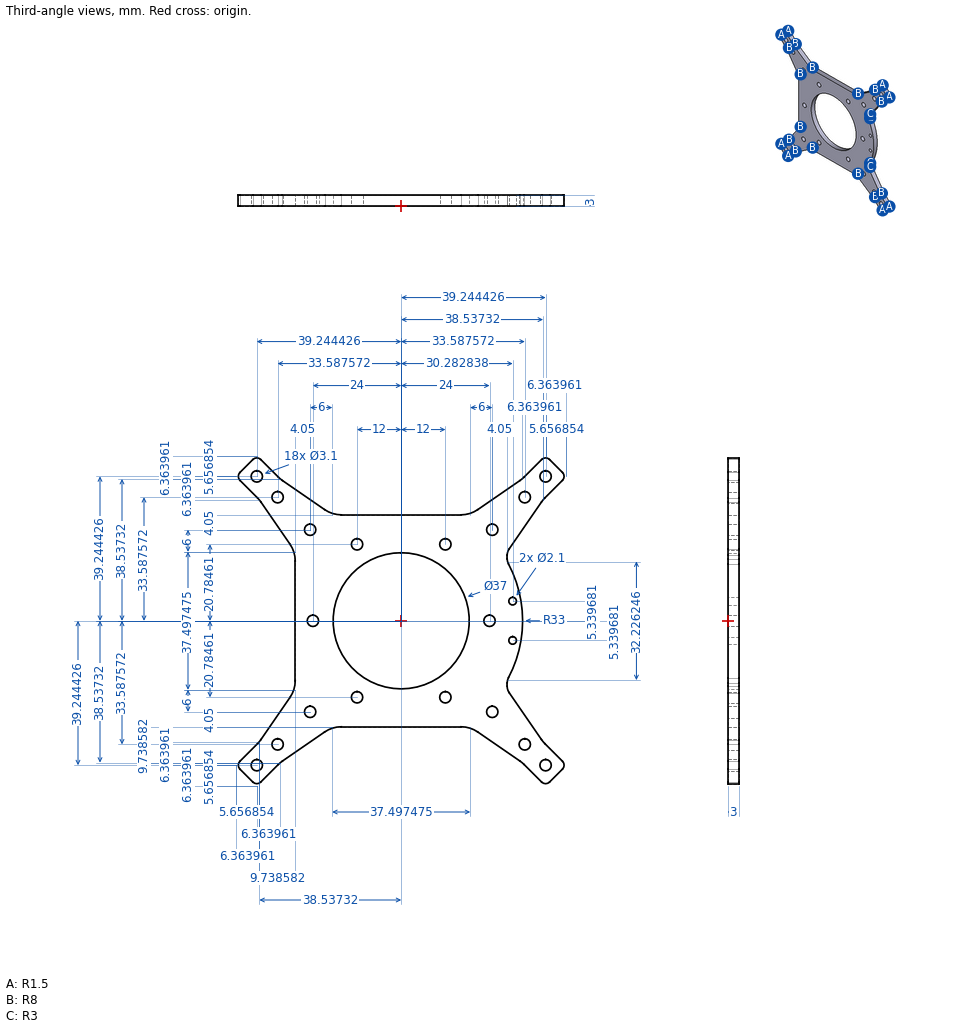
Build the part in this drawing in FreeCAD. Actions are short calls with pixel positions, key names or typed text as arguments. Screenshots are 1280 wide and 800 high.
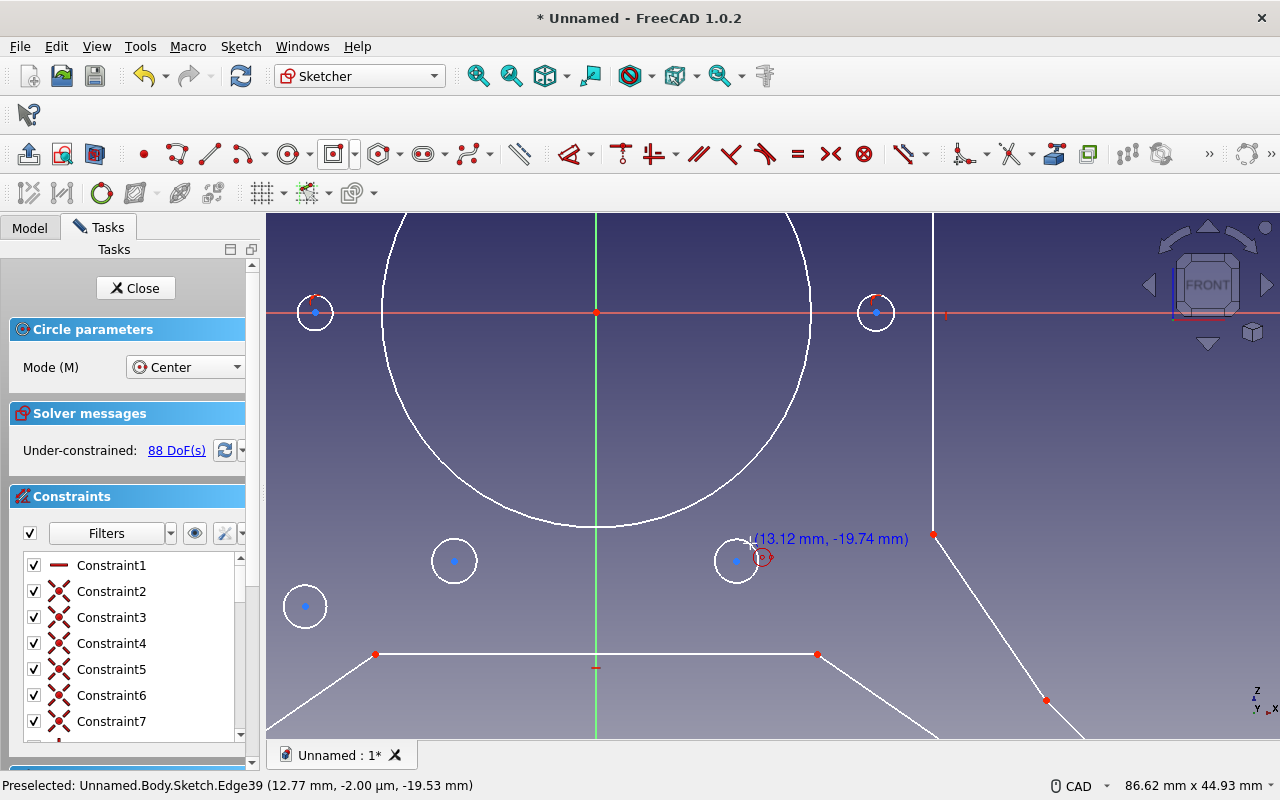
scroll(886, 603, up, 2)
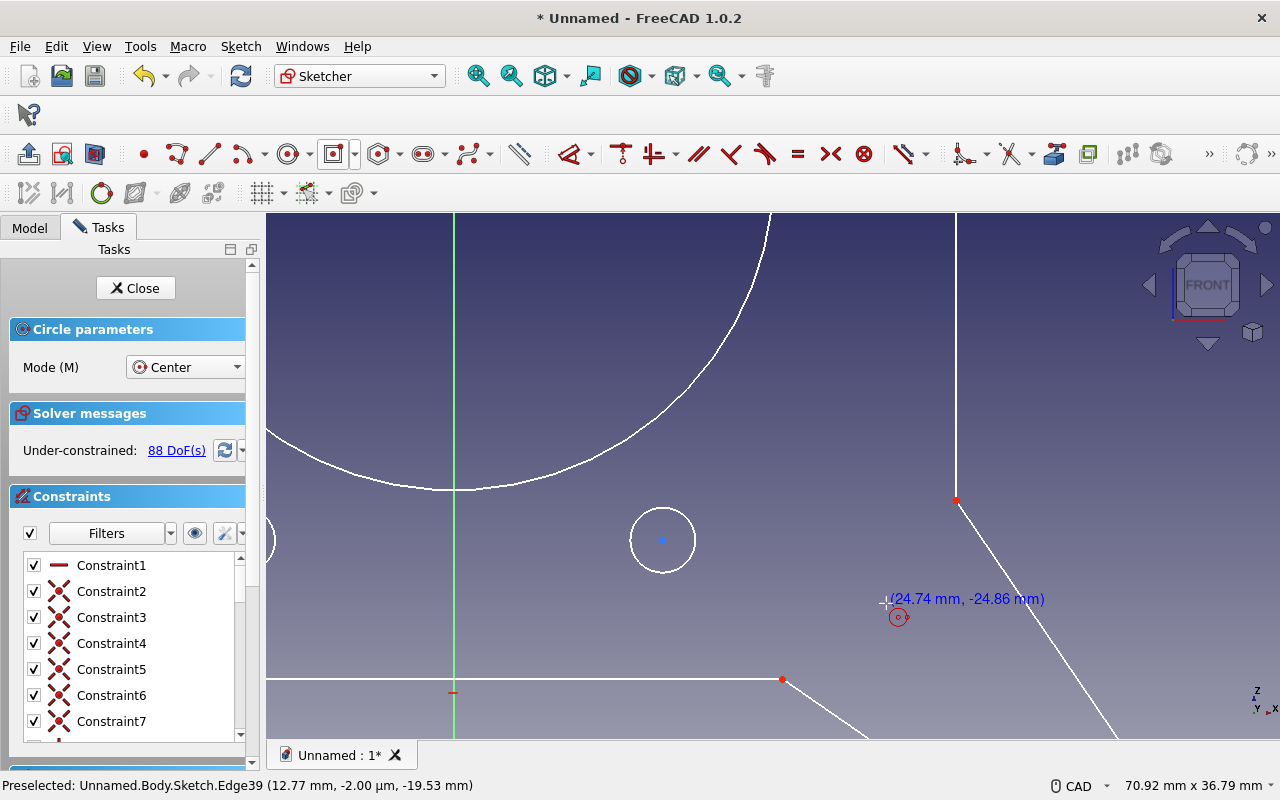
scroll(768, 553, down, 8)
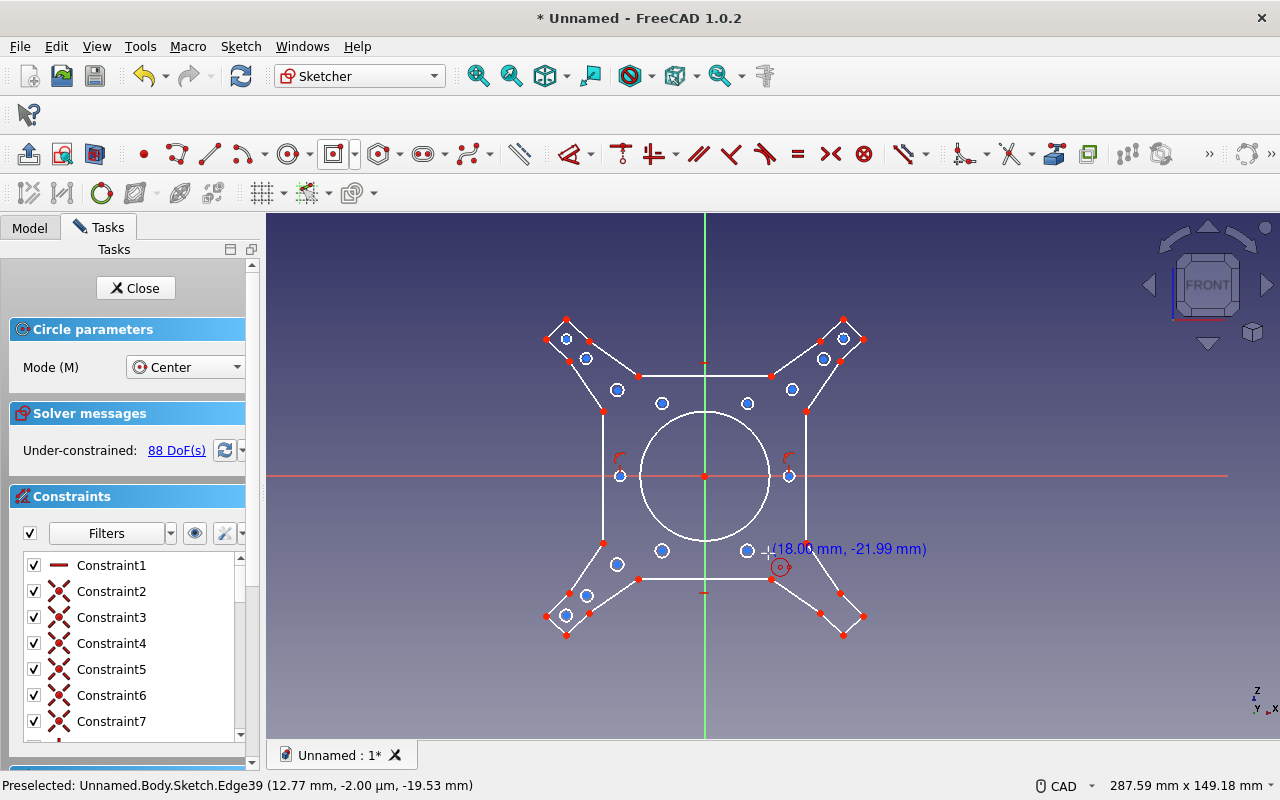
click(792, 563)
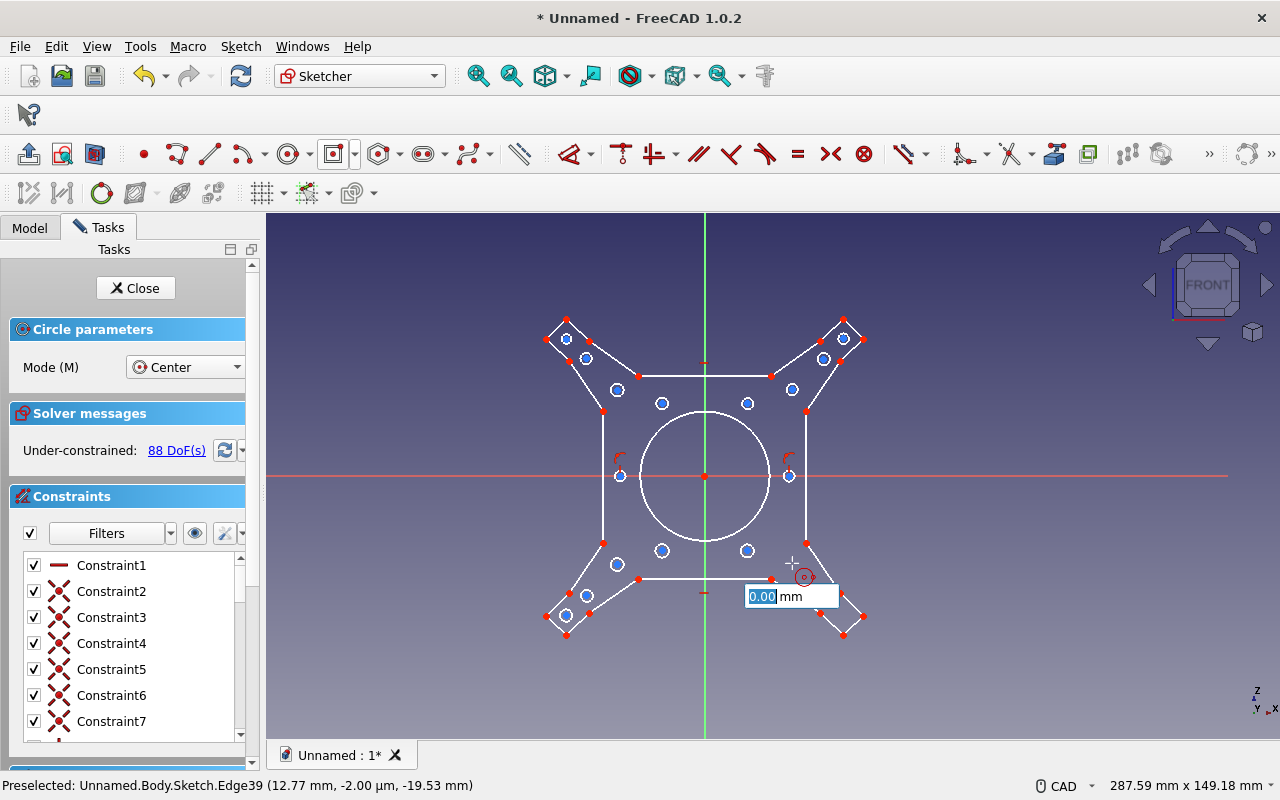
scroll(796, 560, up, 6)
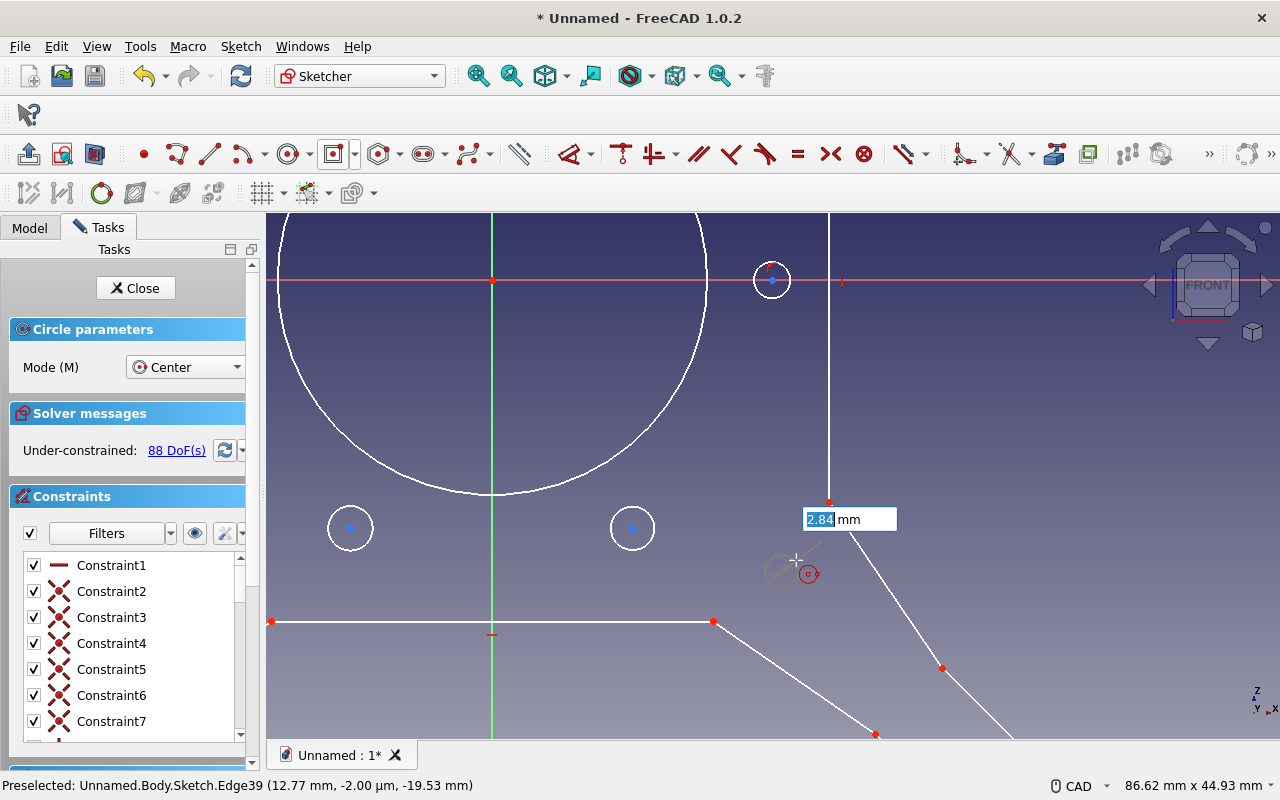
click(795, 557)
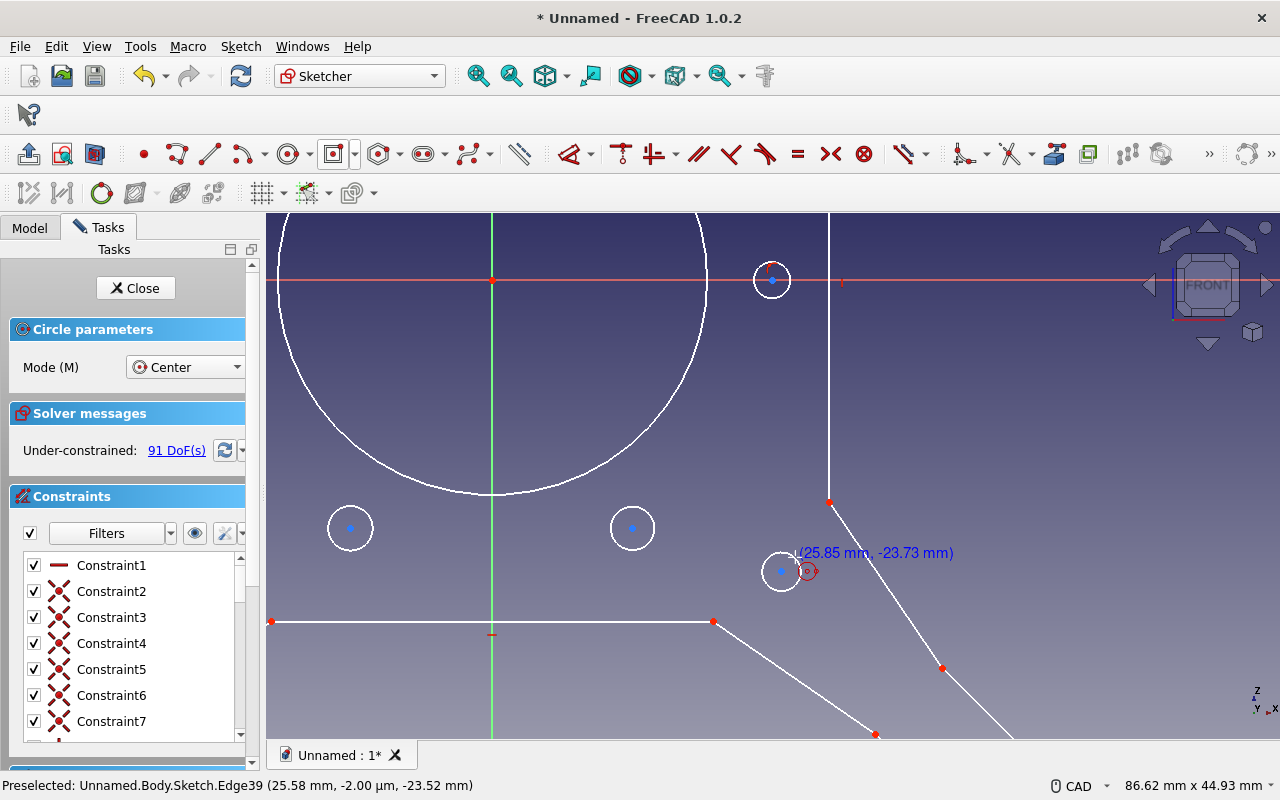
scroll(886, 673, up, 2)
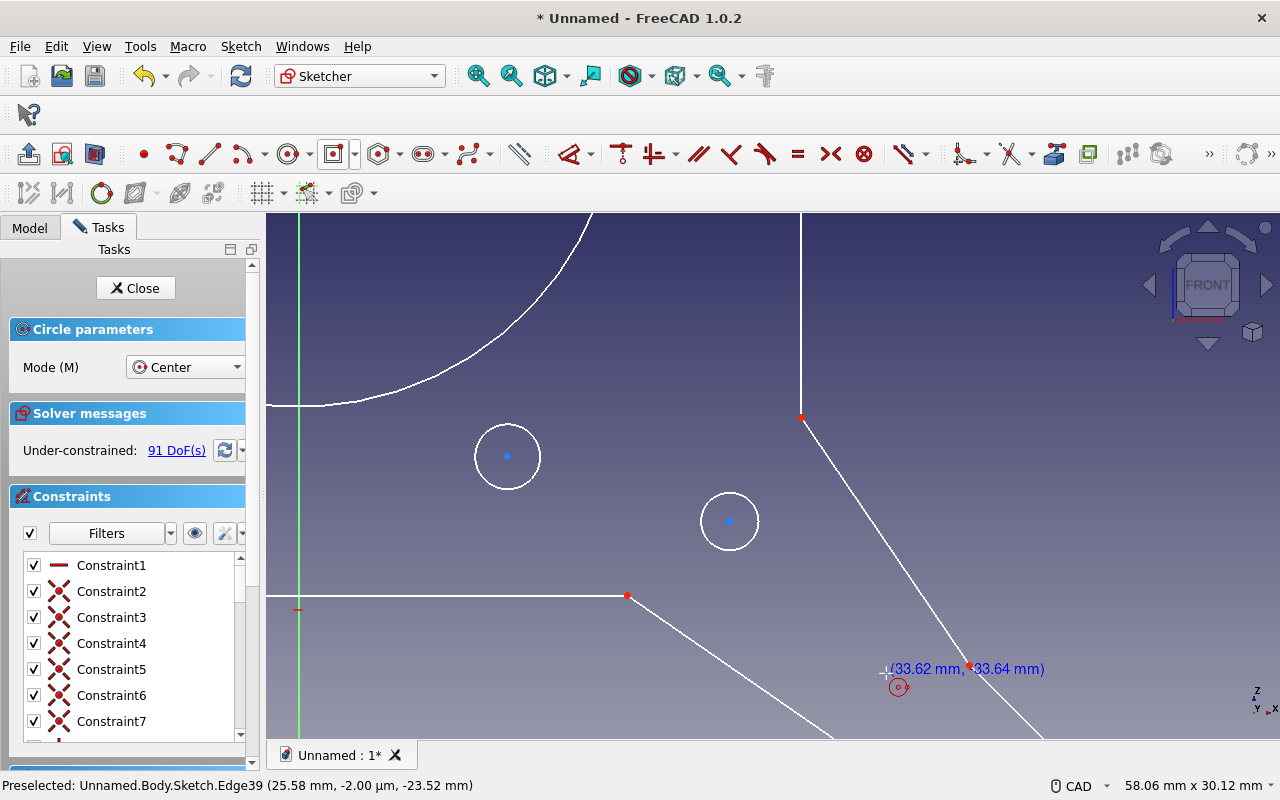
scroll(807, 575, down, 8)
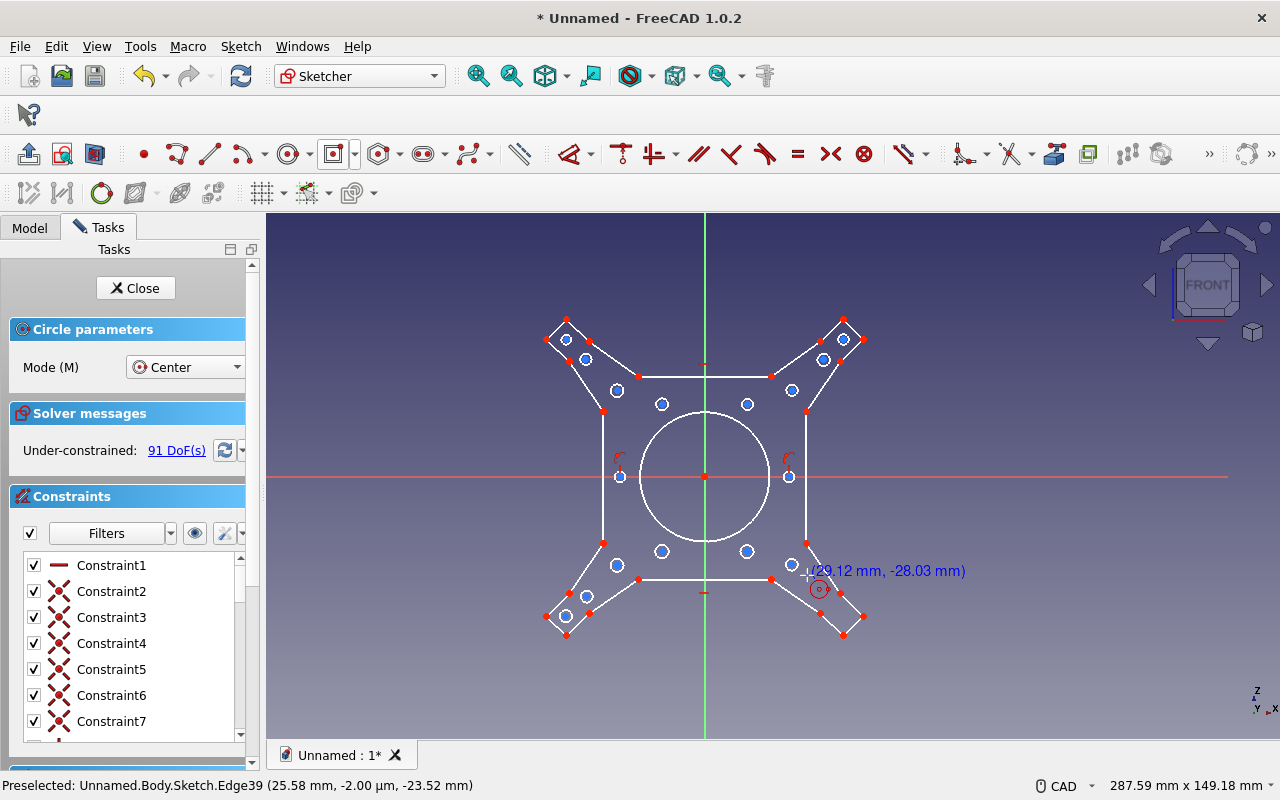
click(823, 595)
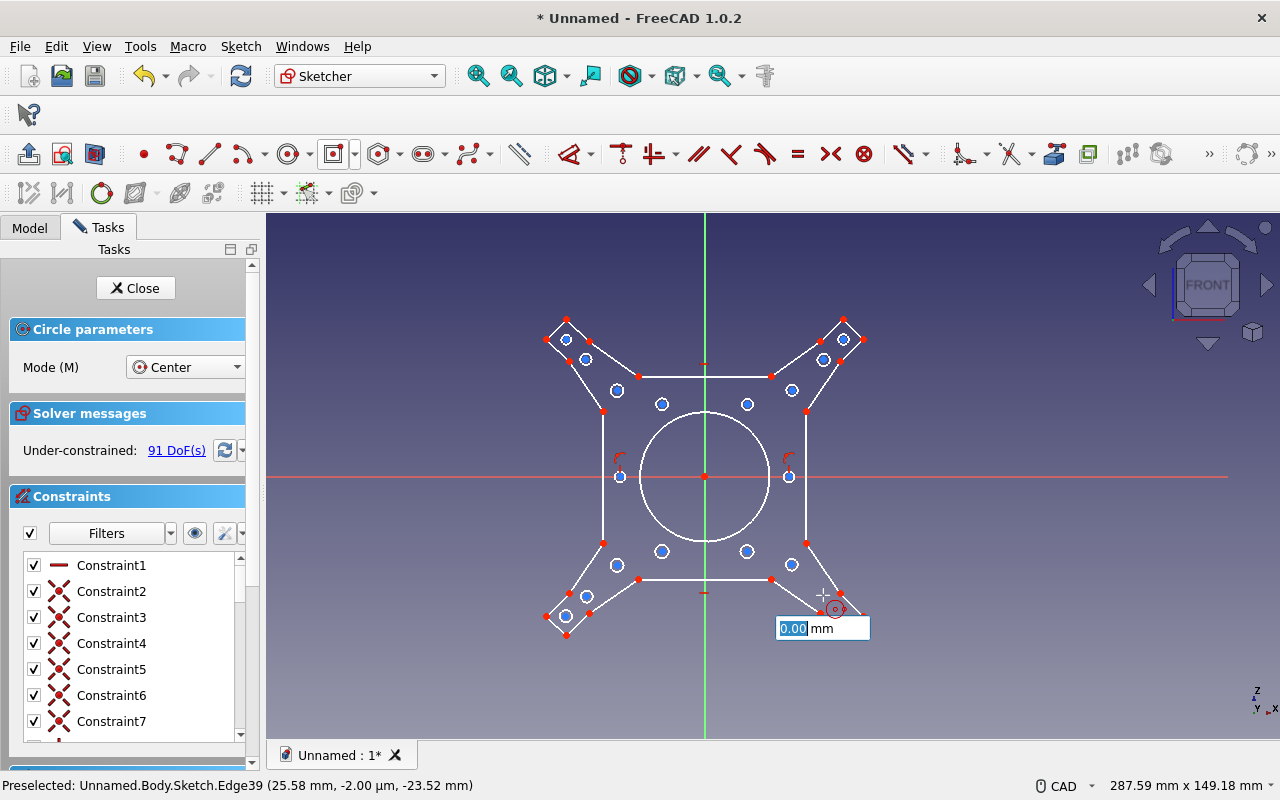
scroll(819, 591, up, 6)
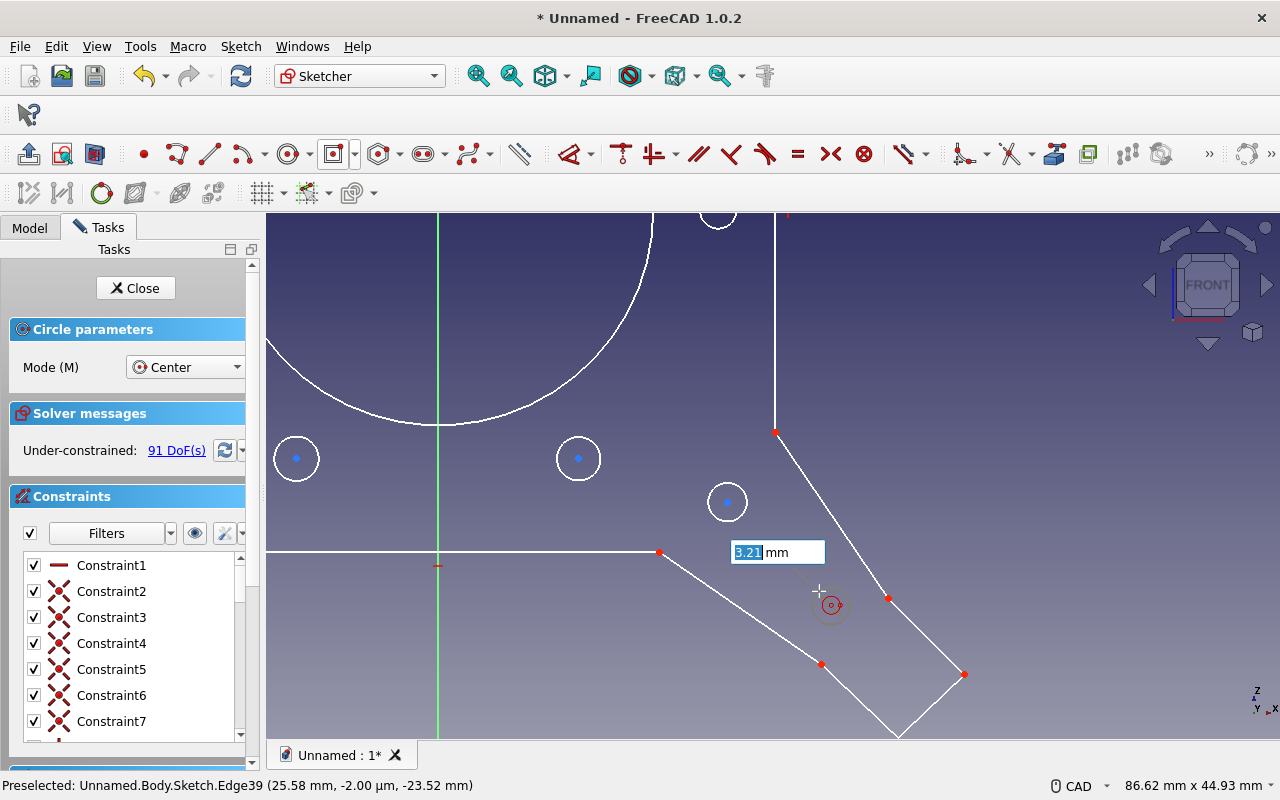
click(819, 591)